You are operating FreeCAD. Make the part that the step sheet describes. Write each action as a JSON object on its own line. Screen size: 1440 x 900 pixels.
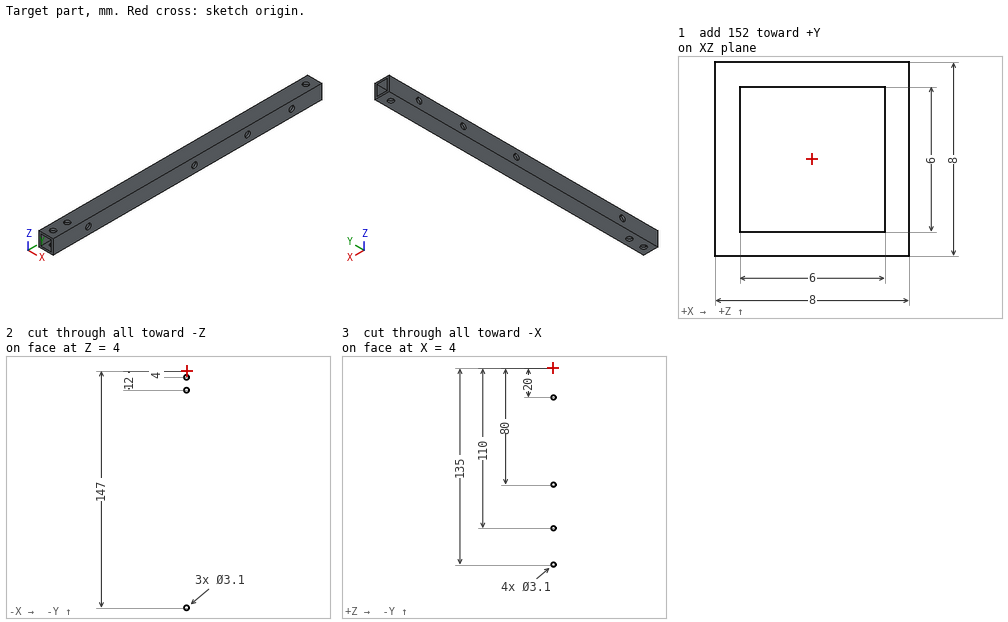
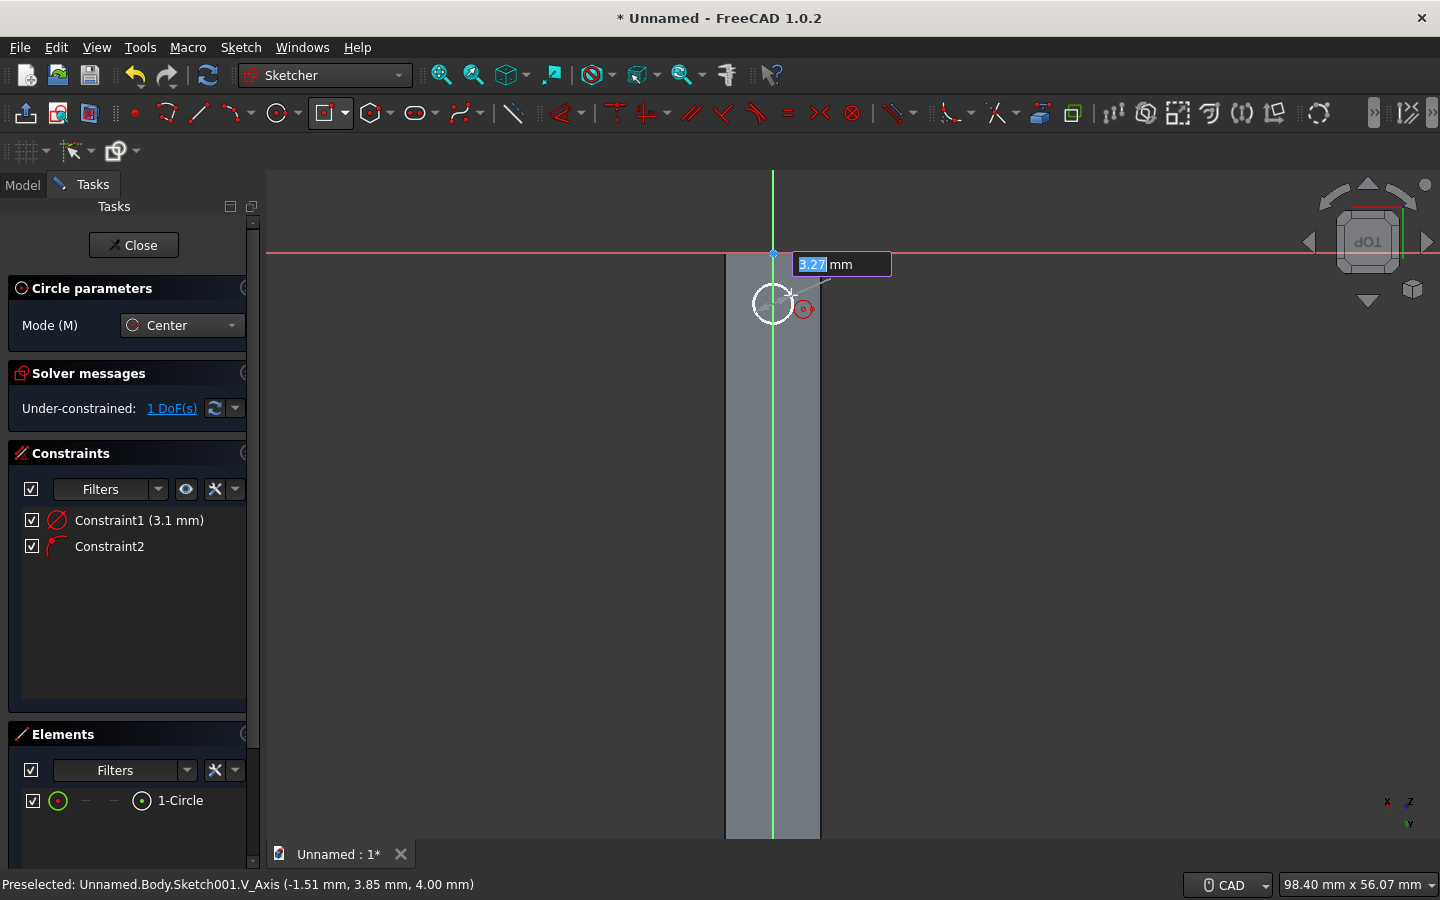
{"action": "type", "text": "3.1"}
{"action": "key", "text": "Return"}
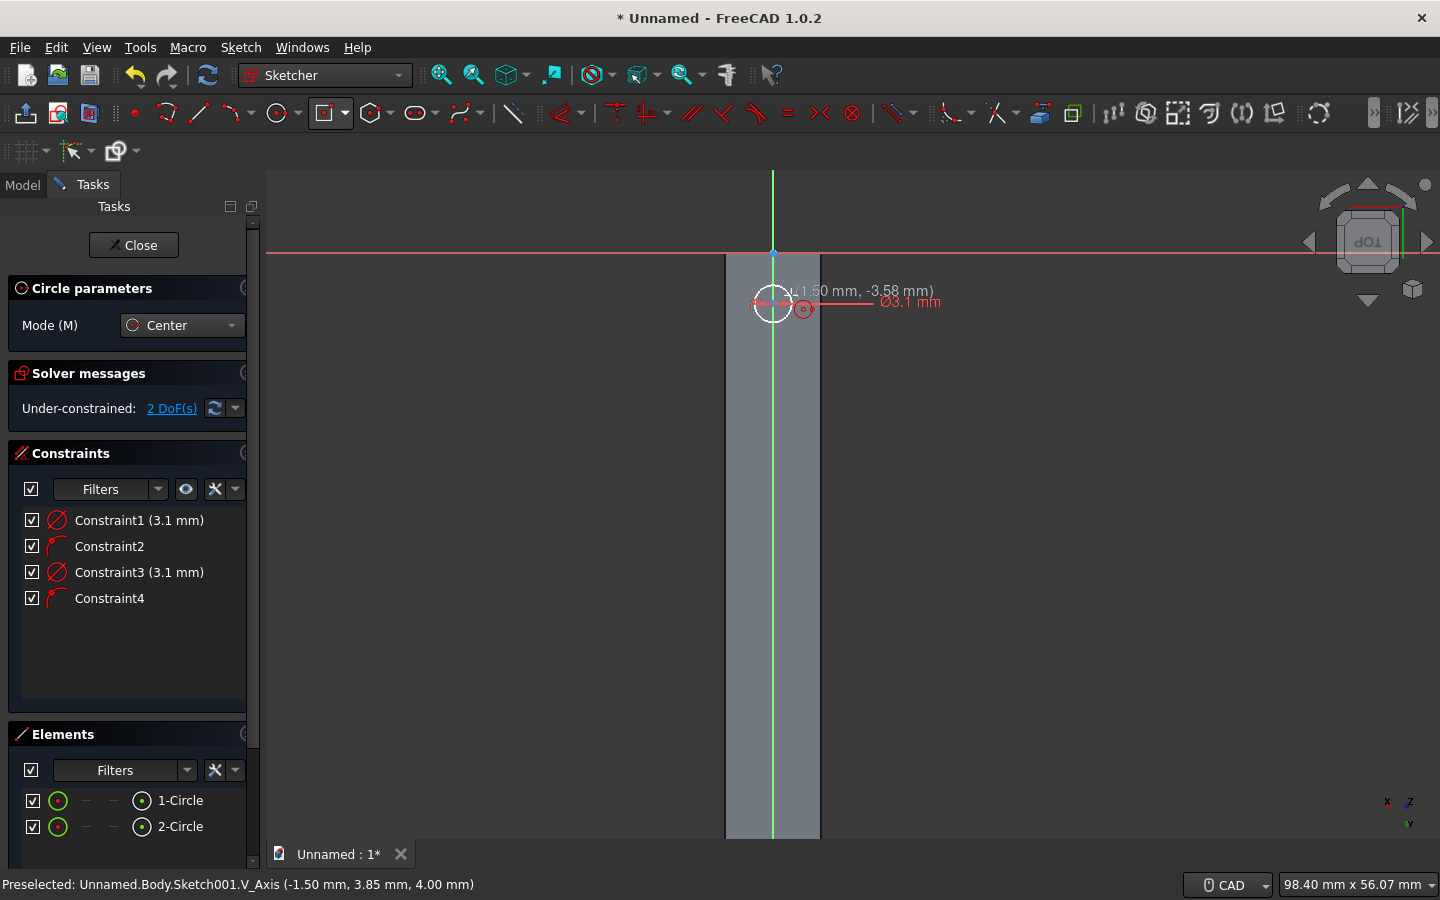
{"action": "scroll", "coordinate": [773, 396], "scroll_direction": "up", "scroll_amount": 2}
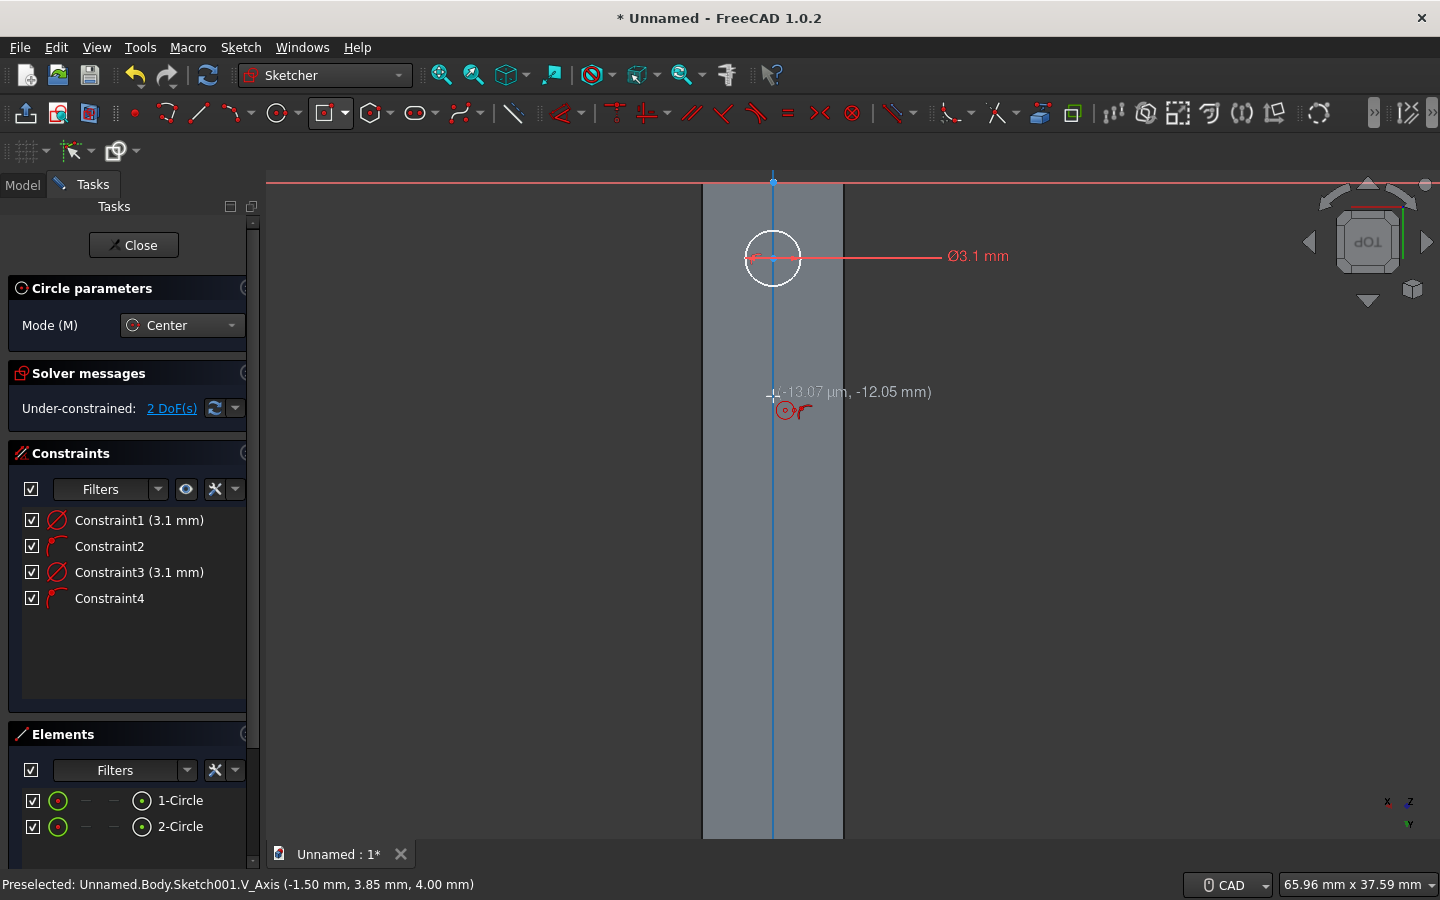
{"action": "scroll", "coordinate": [787, 306], "scroll_direction": "down", "scroll_amount": 9}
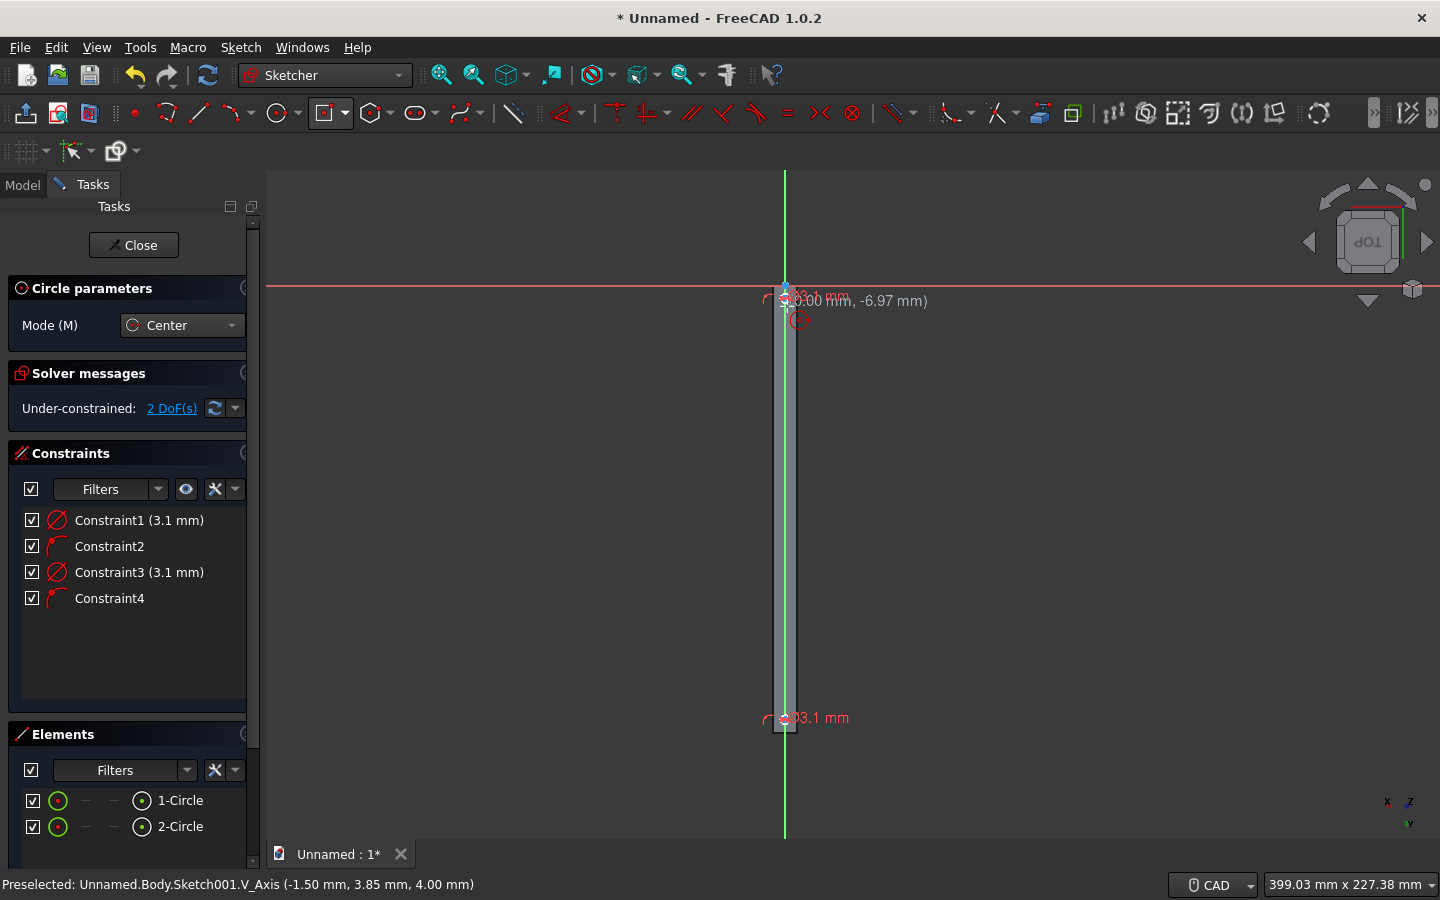
{"action": "left_click", "coordinate": [785, 321]}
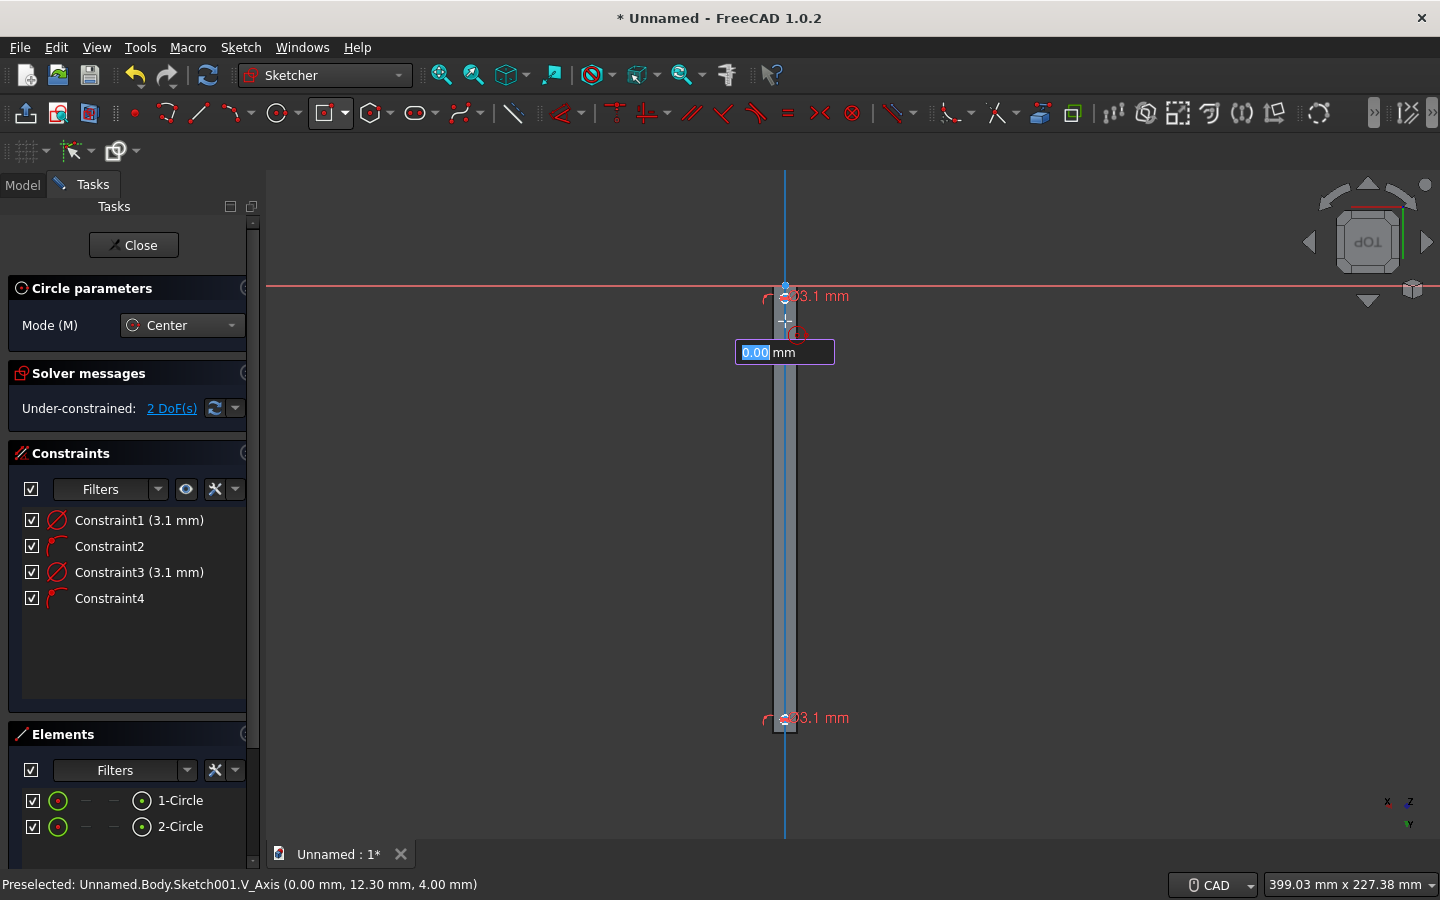
{"action": "scroll", "coordinate": [789, 320], "scroll_direction": "up", "scroll_amount": 7}
{"action": "mouse_move", "coordinate": [789, 318]}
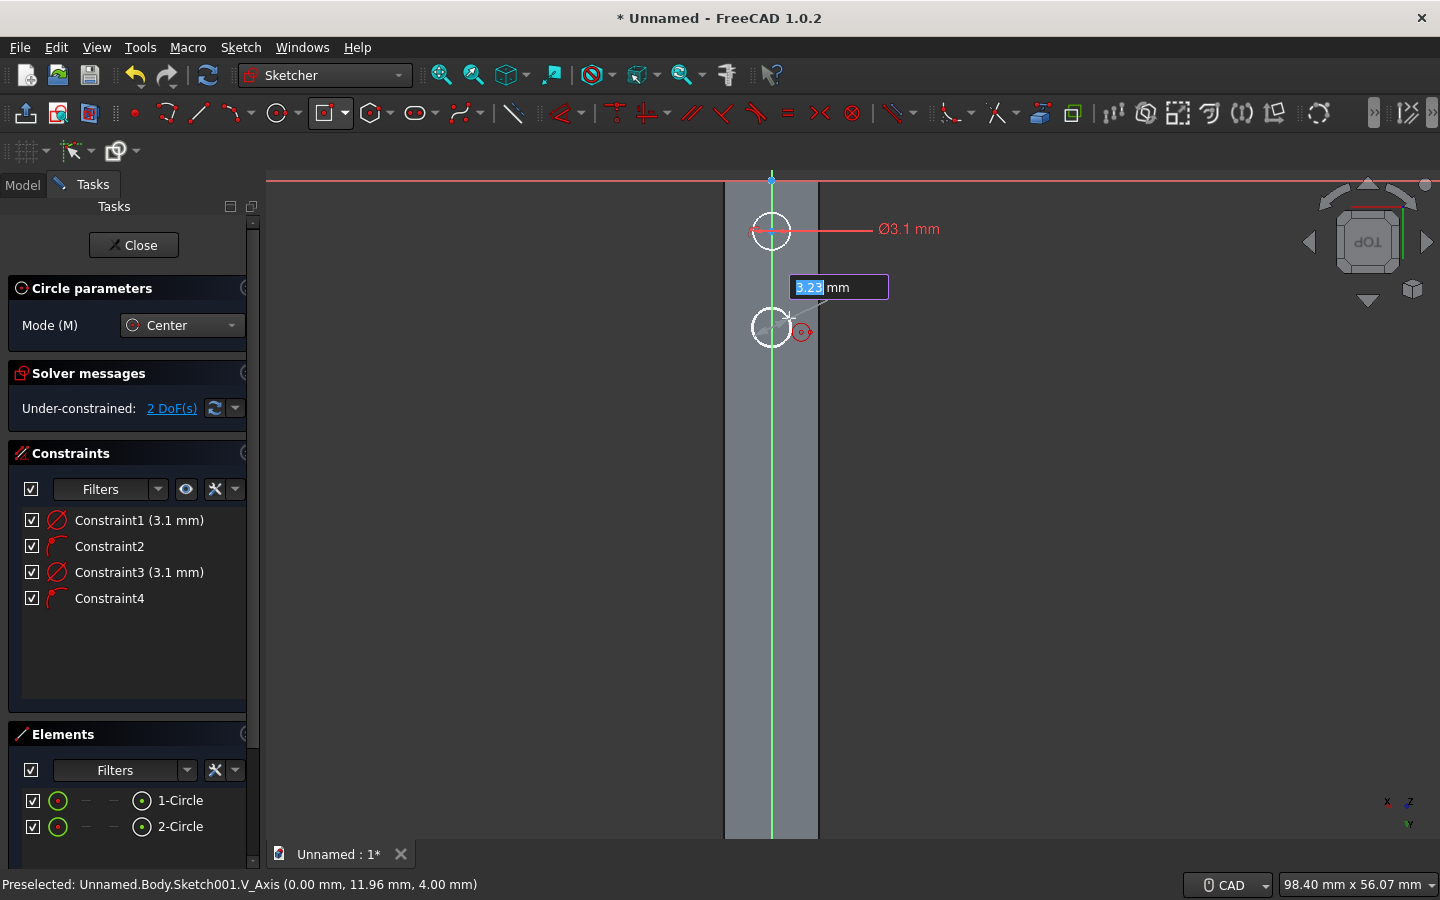
{"action": "type", "text": "3.1"}
{"action": "key", "text": "Return"}
{"action": "key", "text": "Escape"}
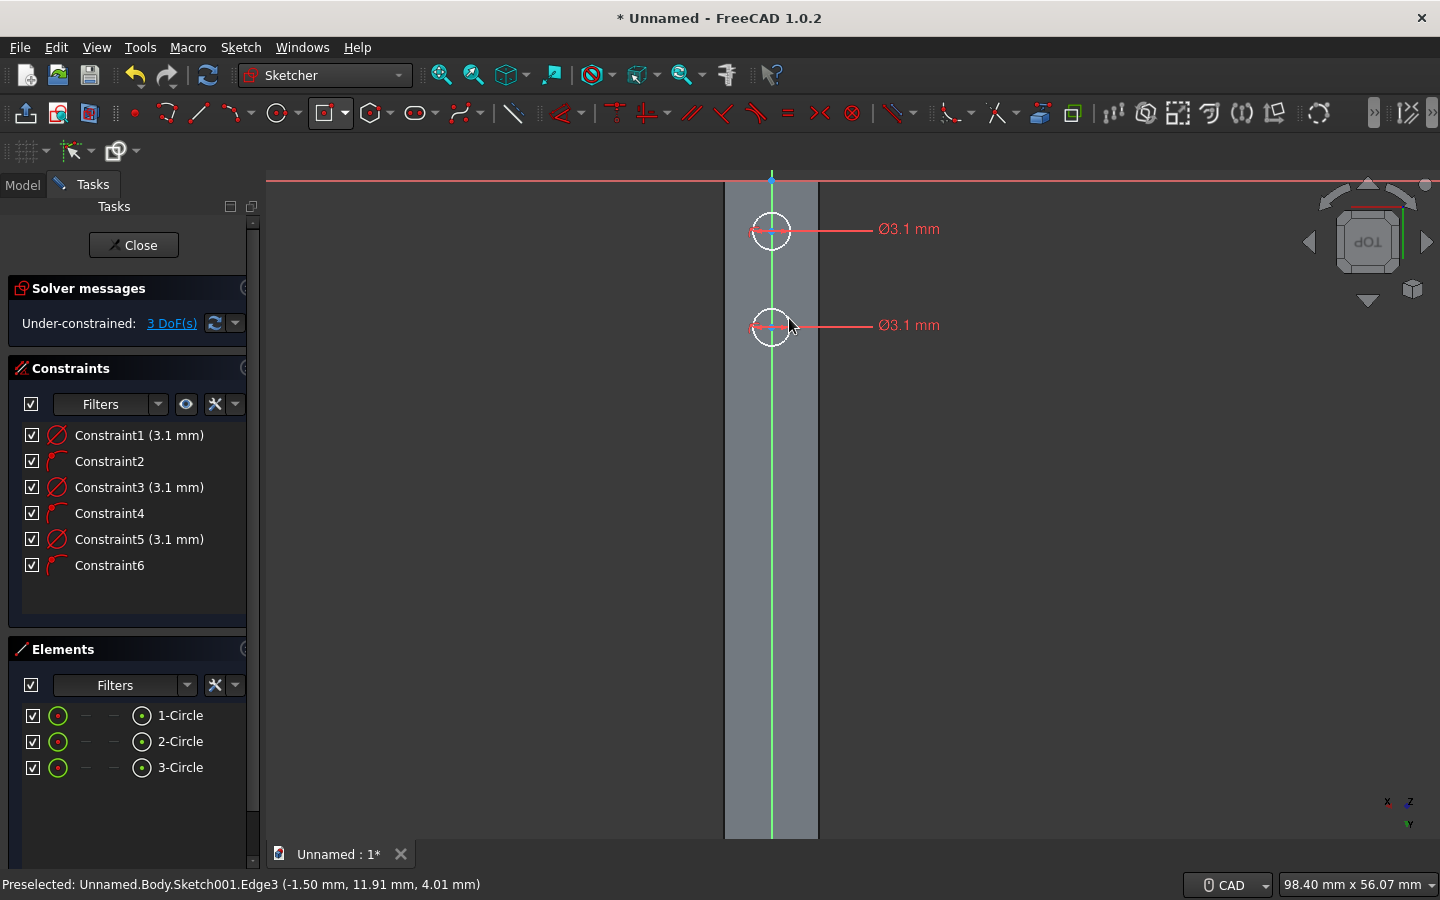
{"action": "left_click", "coordinate": [772, 231]}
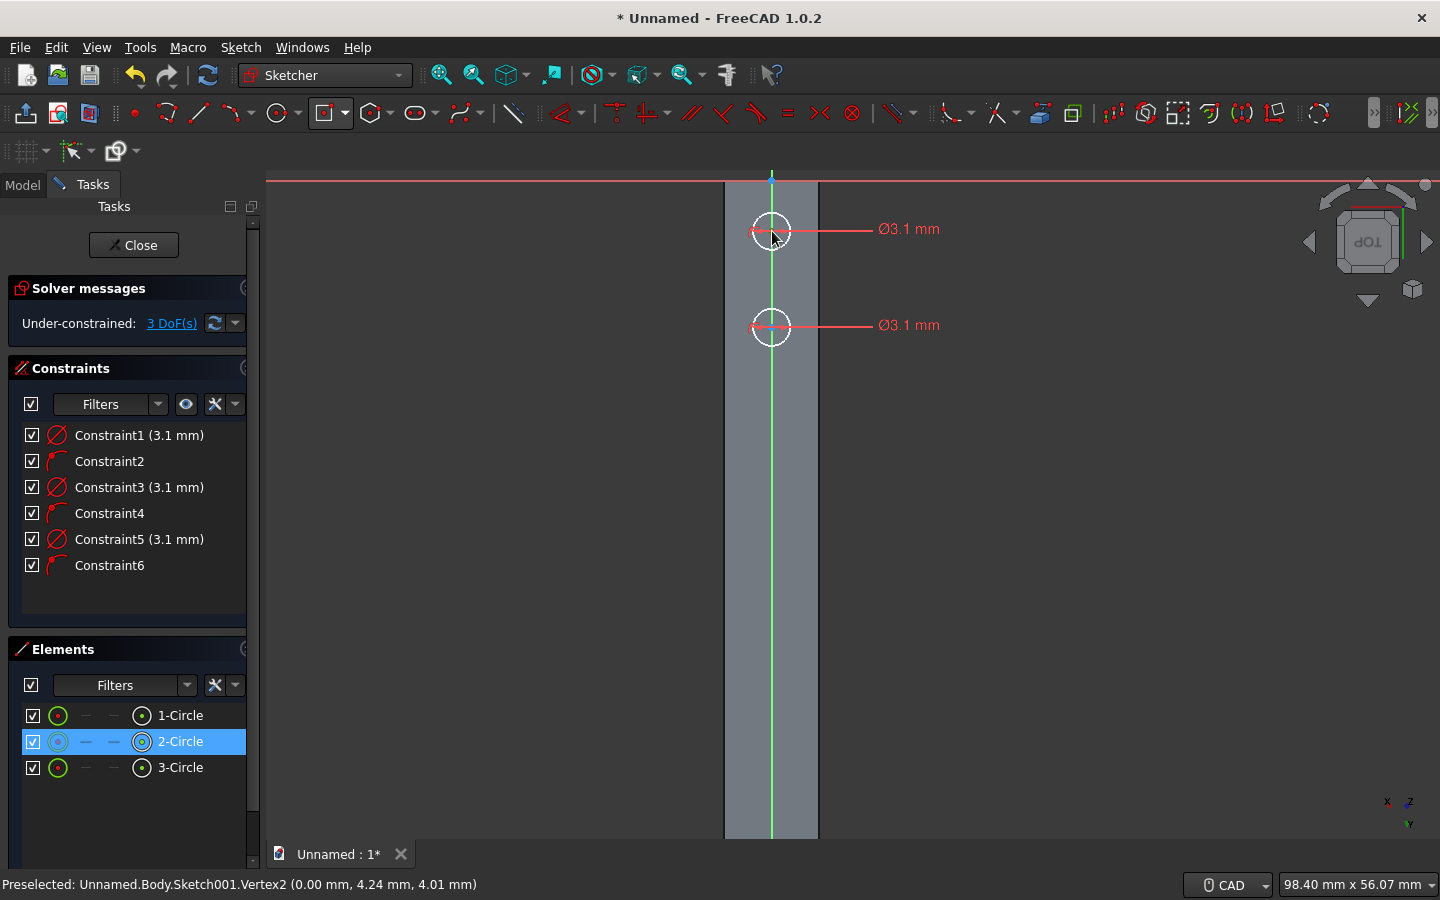
{"action": "left_click", "coordinate": [584, 114]}